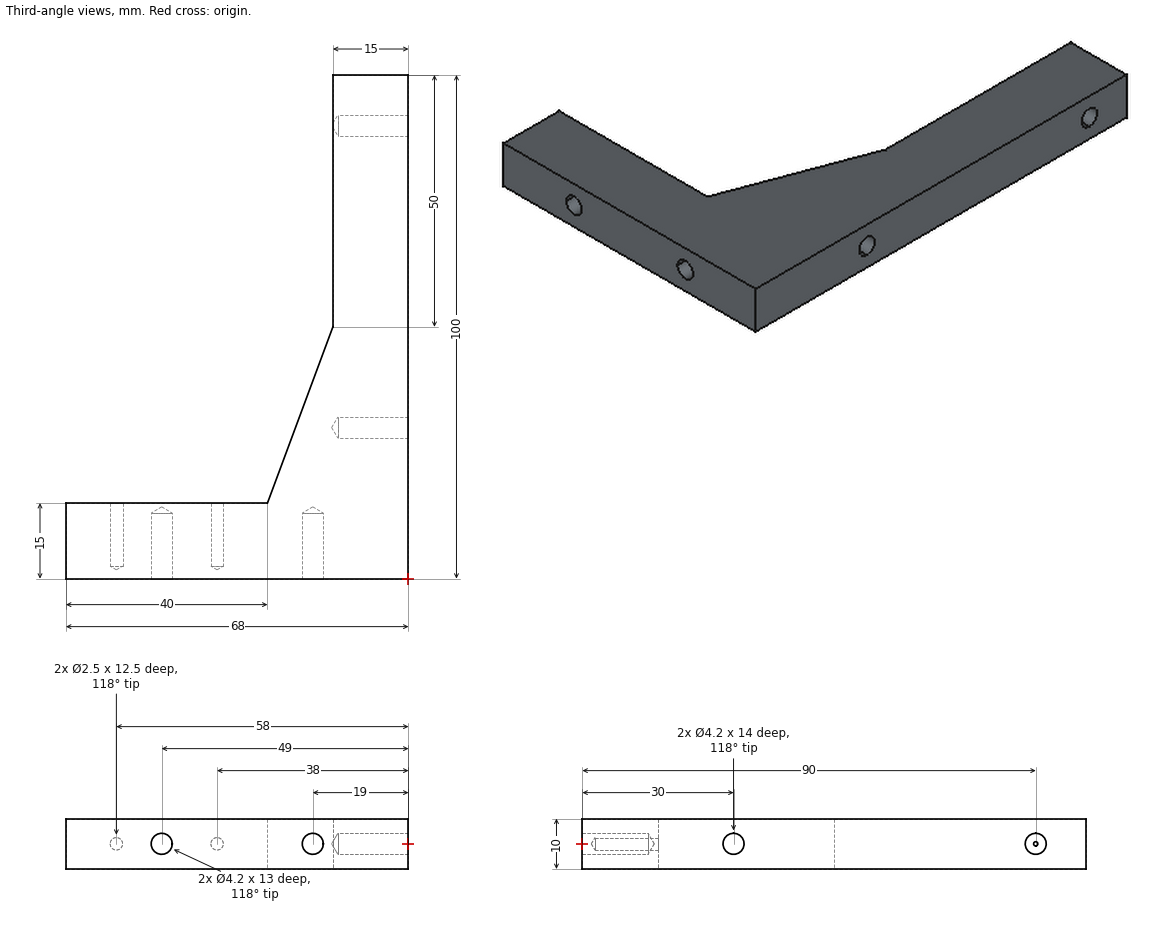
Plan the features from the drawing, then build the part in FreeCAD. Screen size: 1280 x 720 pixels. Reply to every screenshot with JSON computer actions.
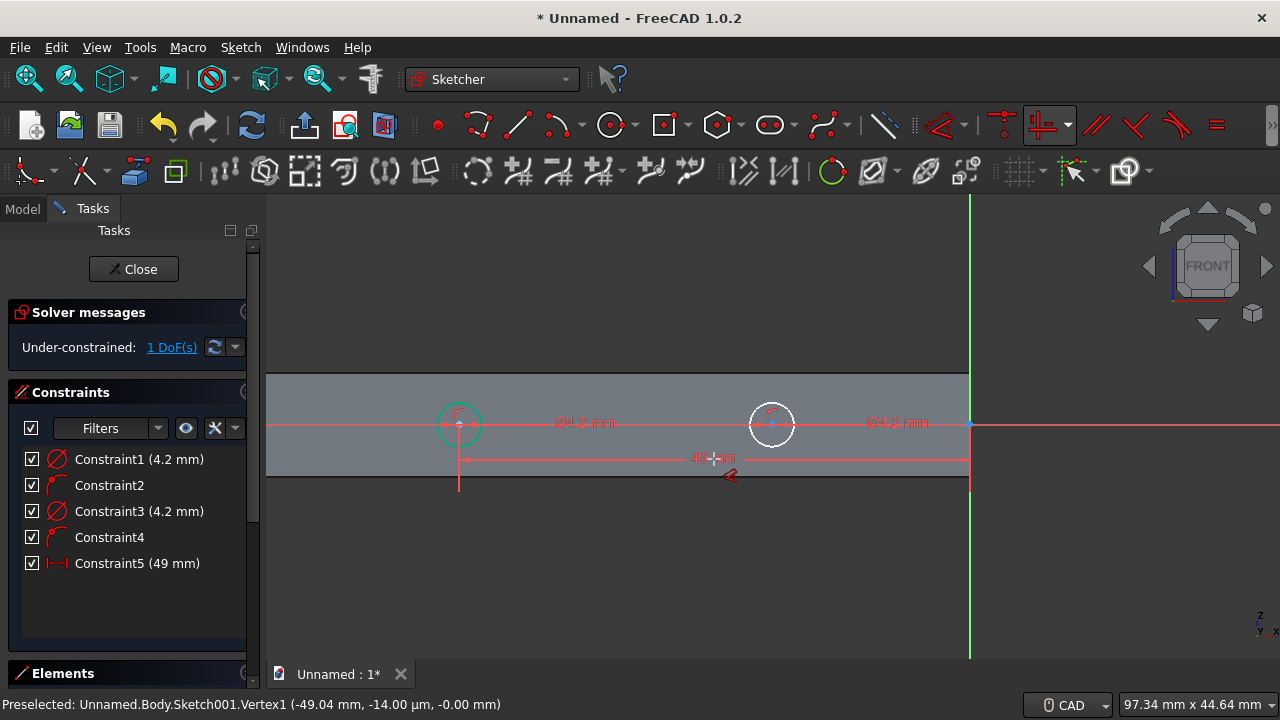
{"action": "left_click", "coordinate": [772, 425]}
{"action": "left_click", "coordinate": [871, 459]}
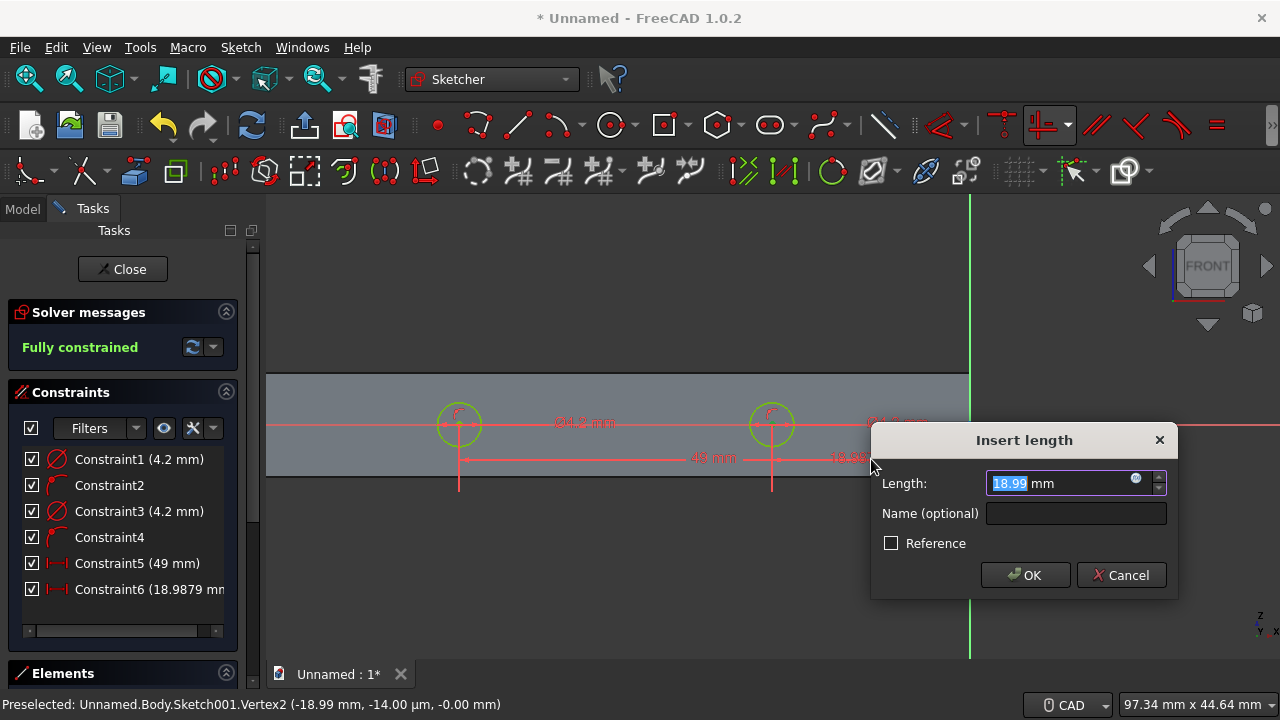
{"action": "type", "text": "19"}
{"action": "key", "text": "Return"}
{"action": "key", "text": "Escape"}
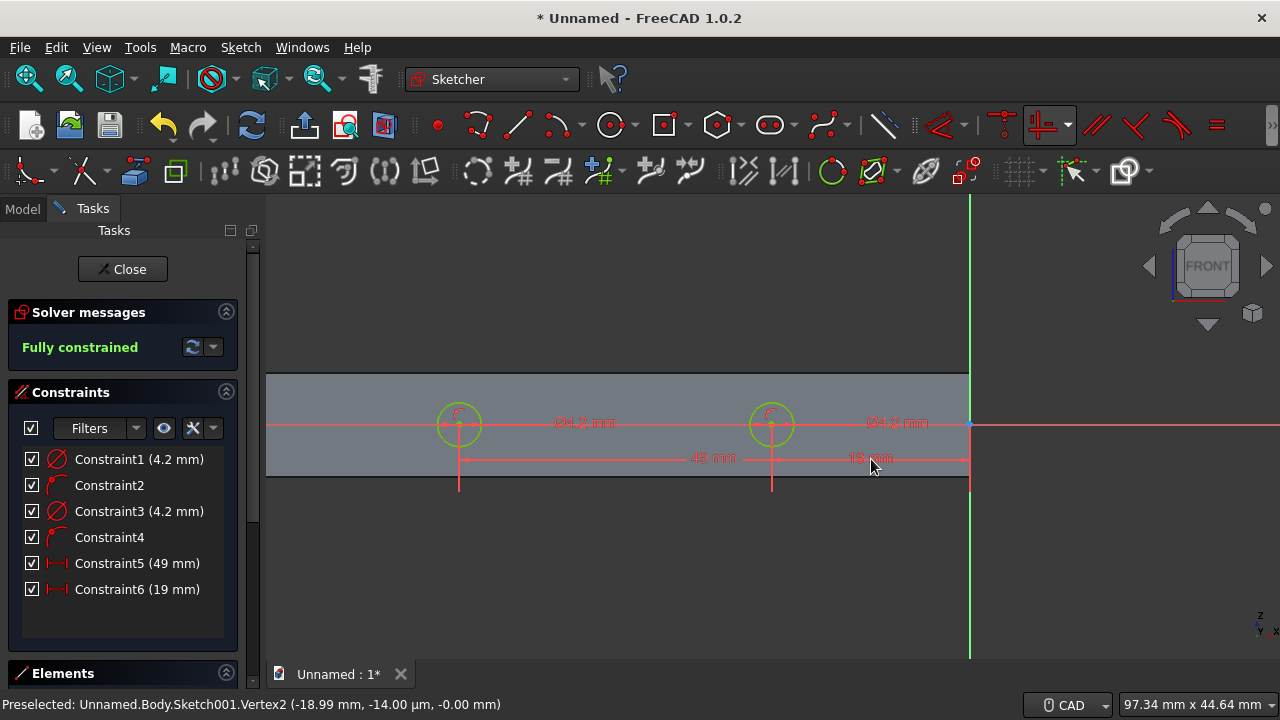
{"action": "left_click", "coordinate": [123, 269]}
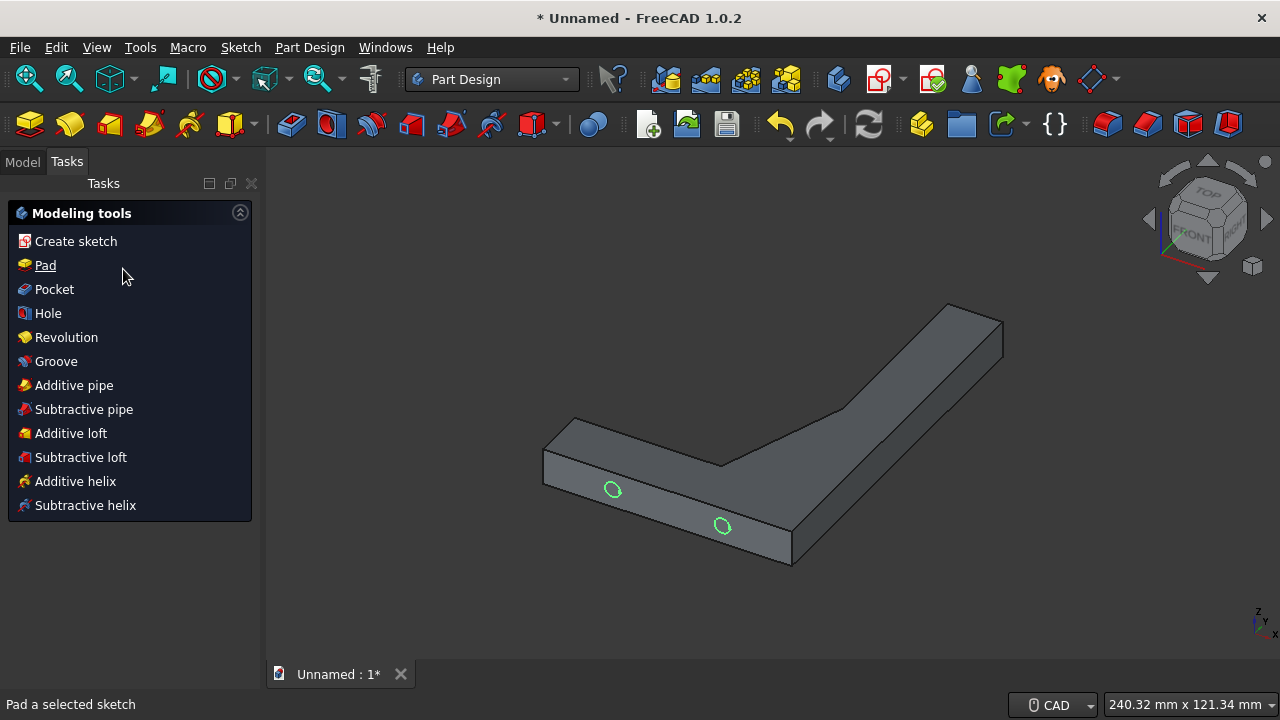
{"action": "left_click", "coordinate": [332, 124]}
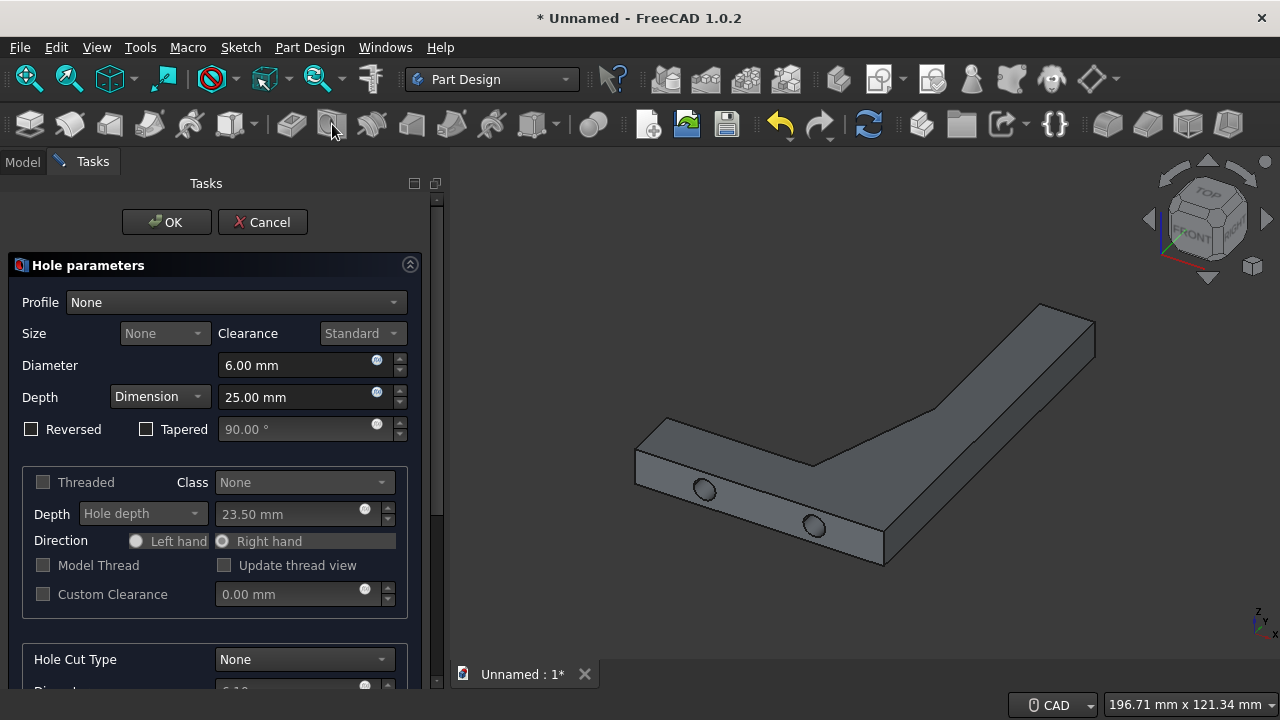
{"action": "triple_click", "coordinate": [305, 365]}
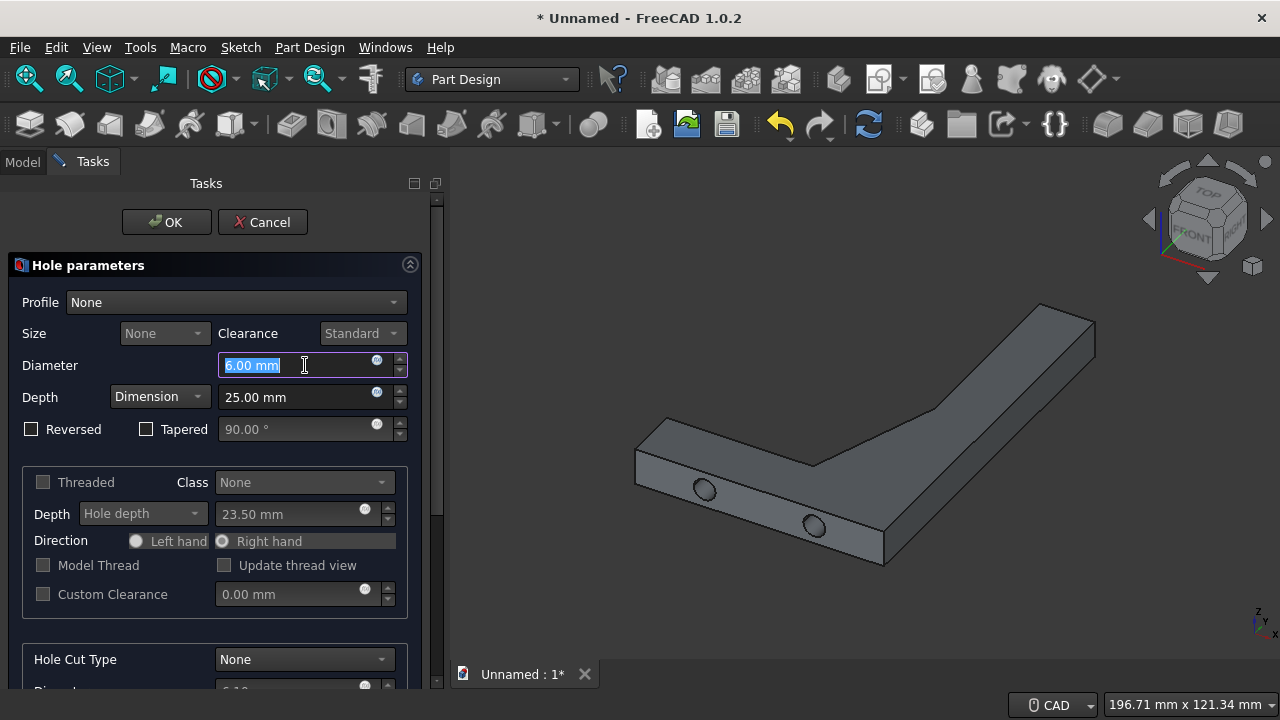
{"action": "type", "text": "4.2"}
{"action": "key", "text": "Tab"}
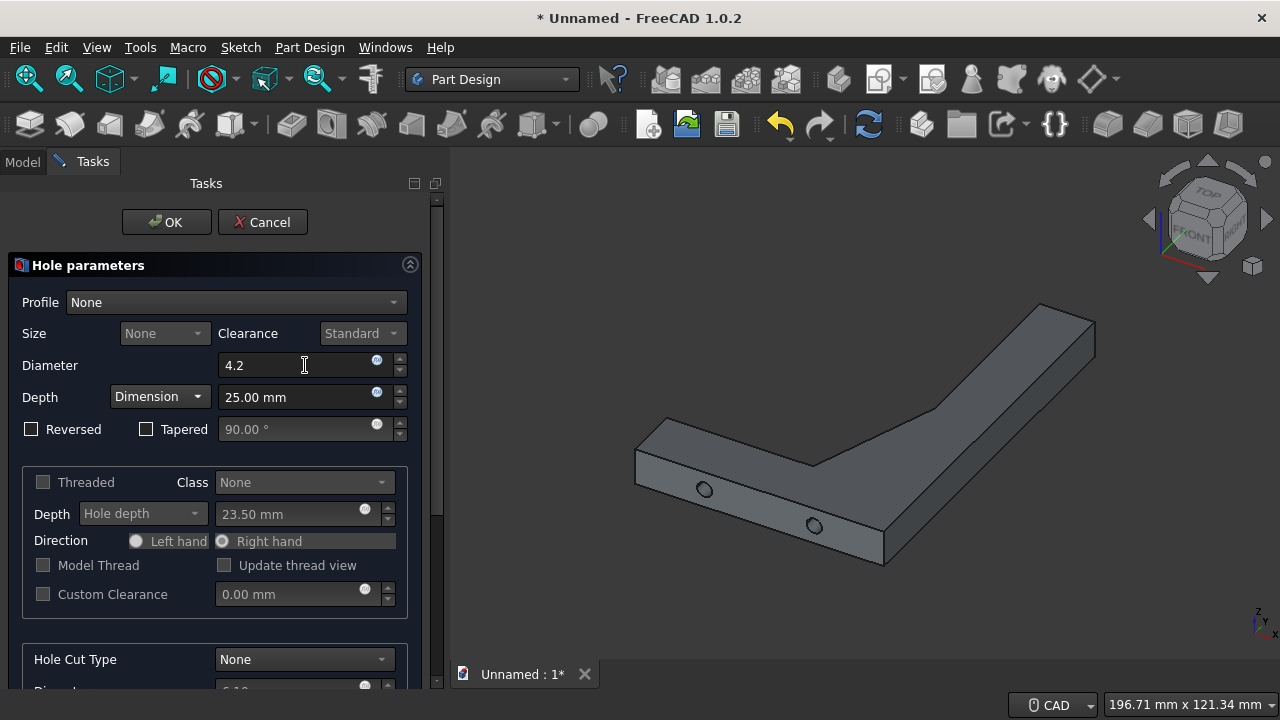
{"action": "triple_click", "coordinate": [305, 397]}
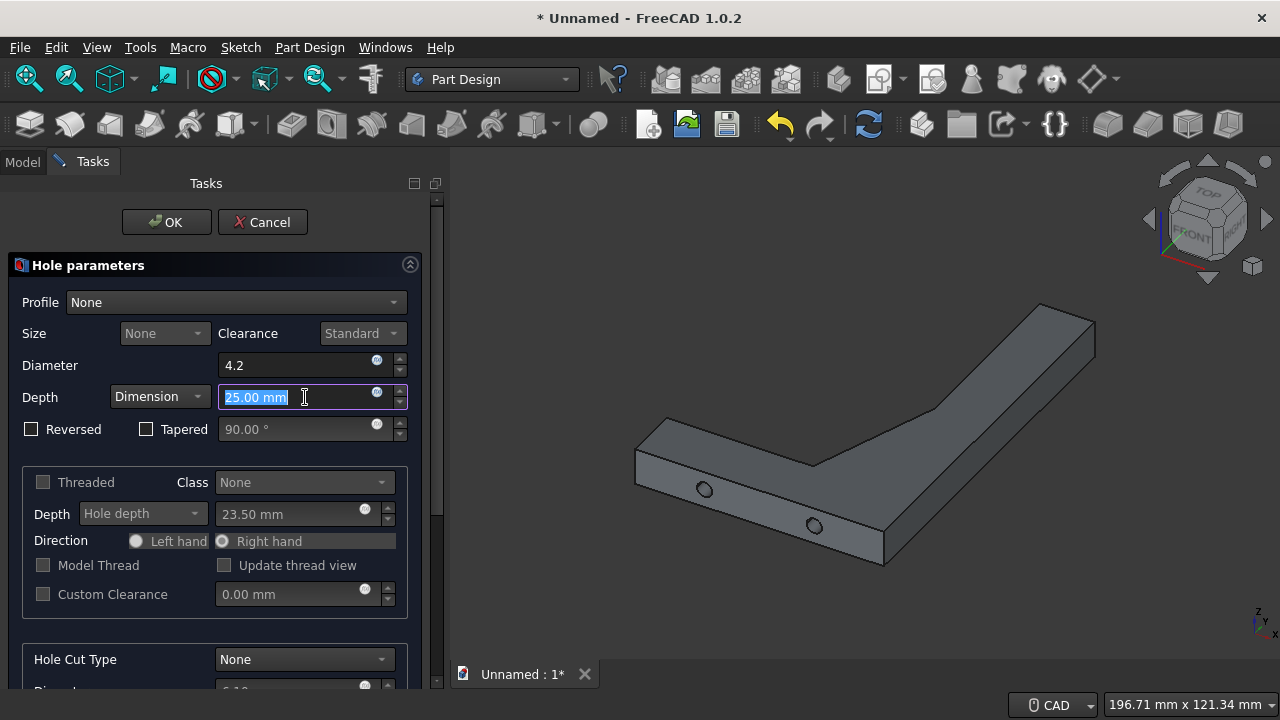
{"action": "type", "text": "13"}
{"action": "key", "text": "Tab"}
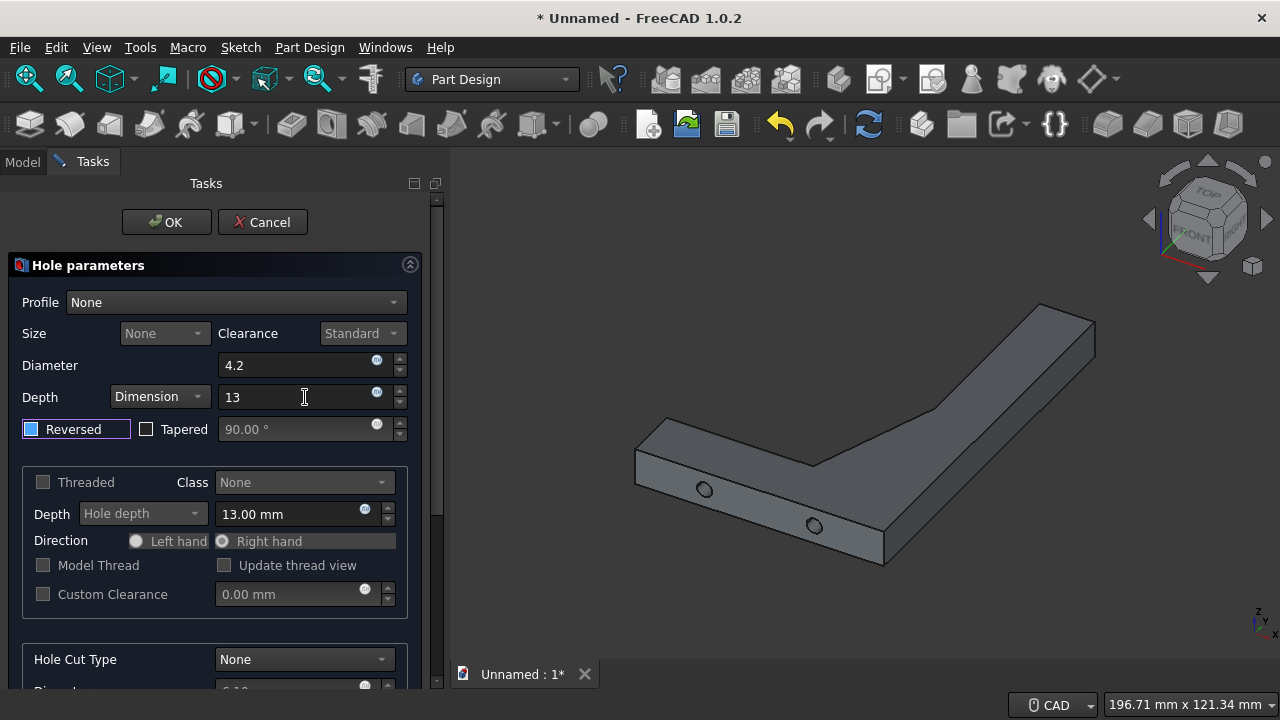
{"action": "left_click", "coordinate": [167, 222]}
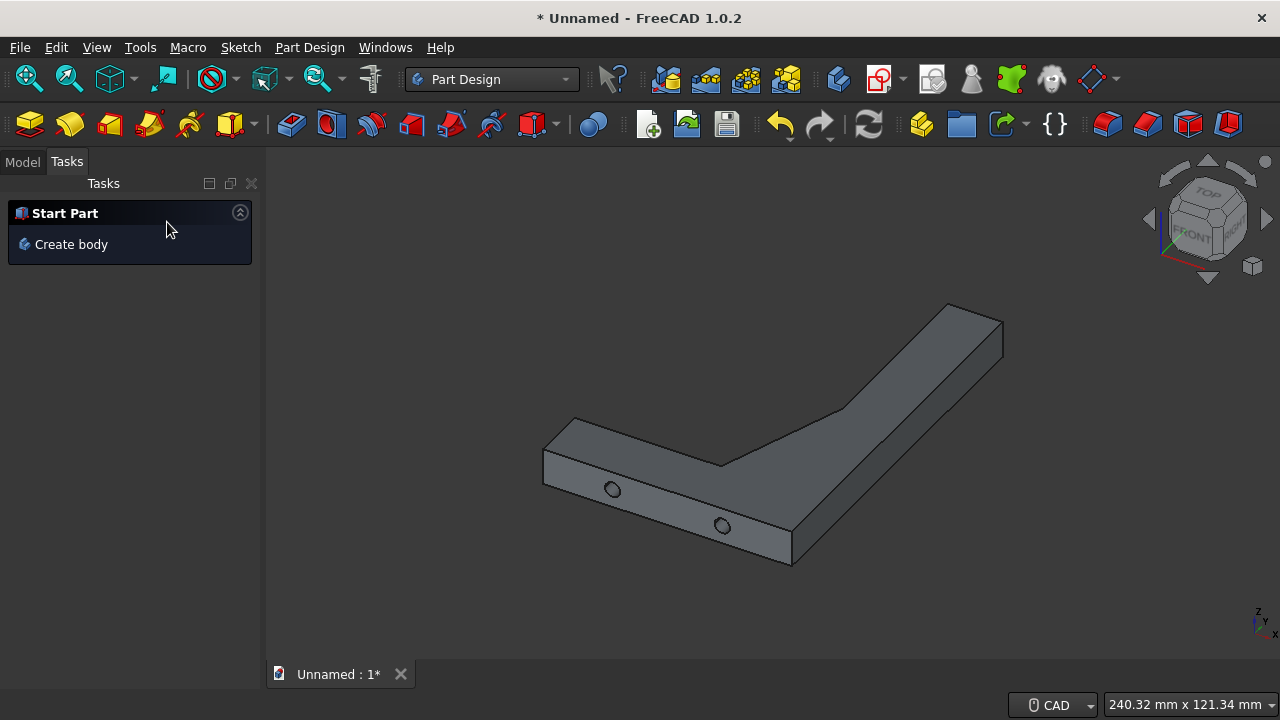
{"action": "left_click", "coordinate": [988, 353]}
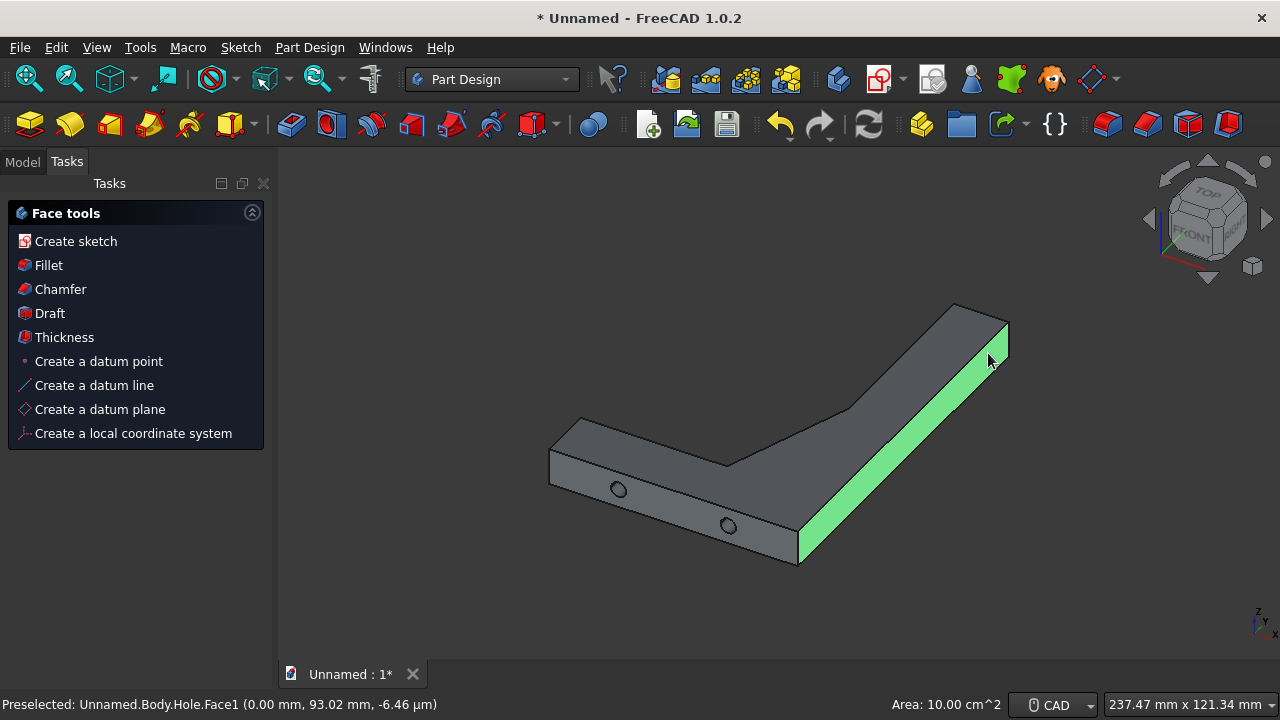
{"action": "left_click", "coordinate": [880, 80]}